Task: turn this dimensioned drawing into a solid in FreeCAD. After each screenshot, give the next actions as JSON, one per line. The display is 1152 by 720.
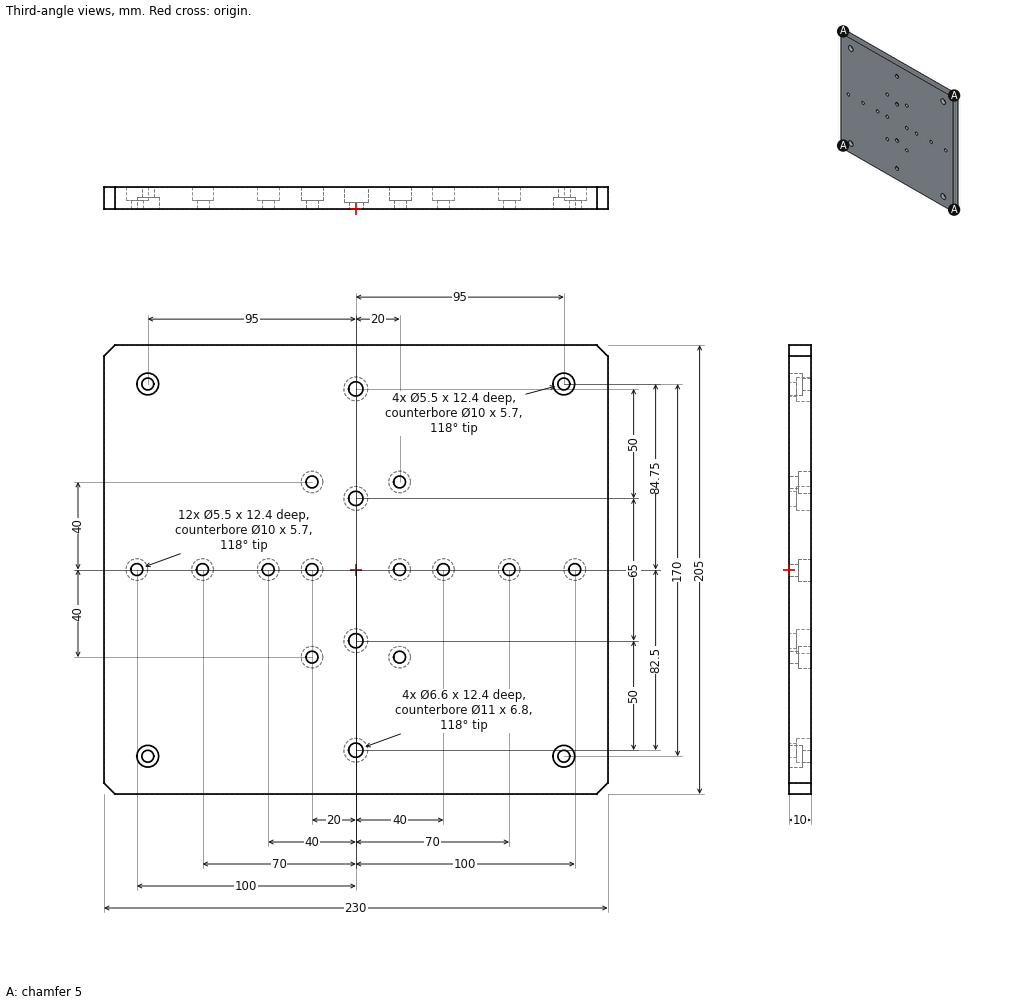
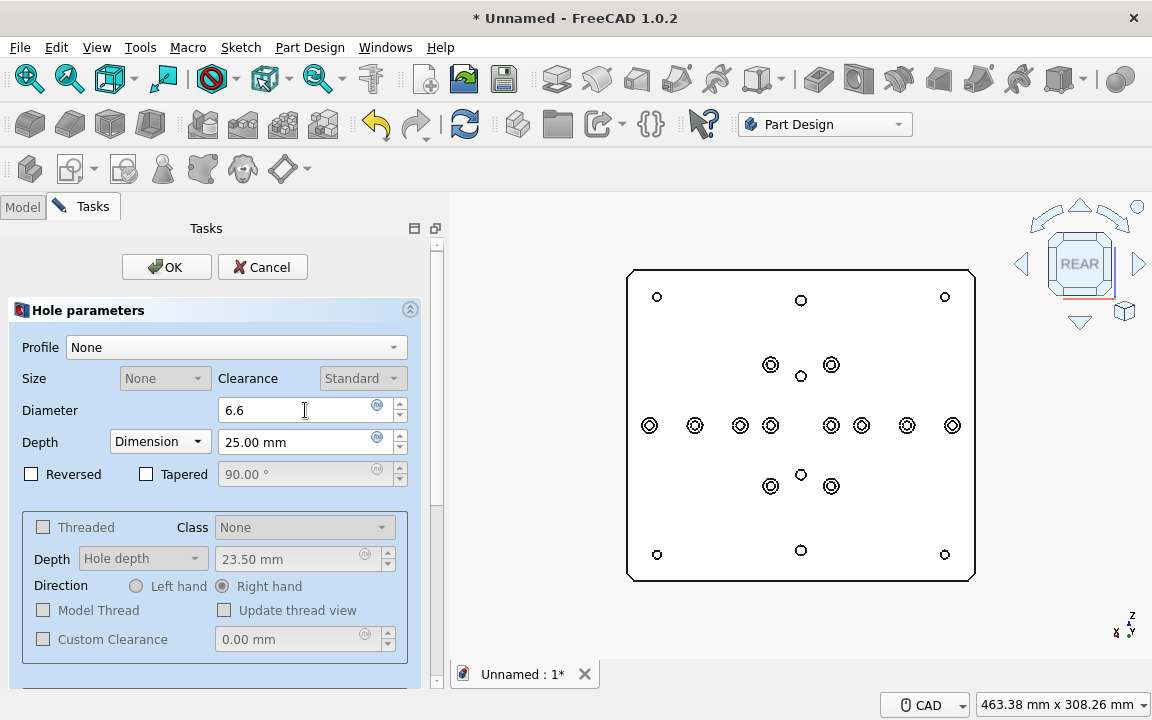
{"action": "triple_click", "coordinate": [305, 442]}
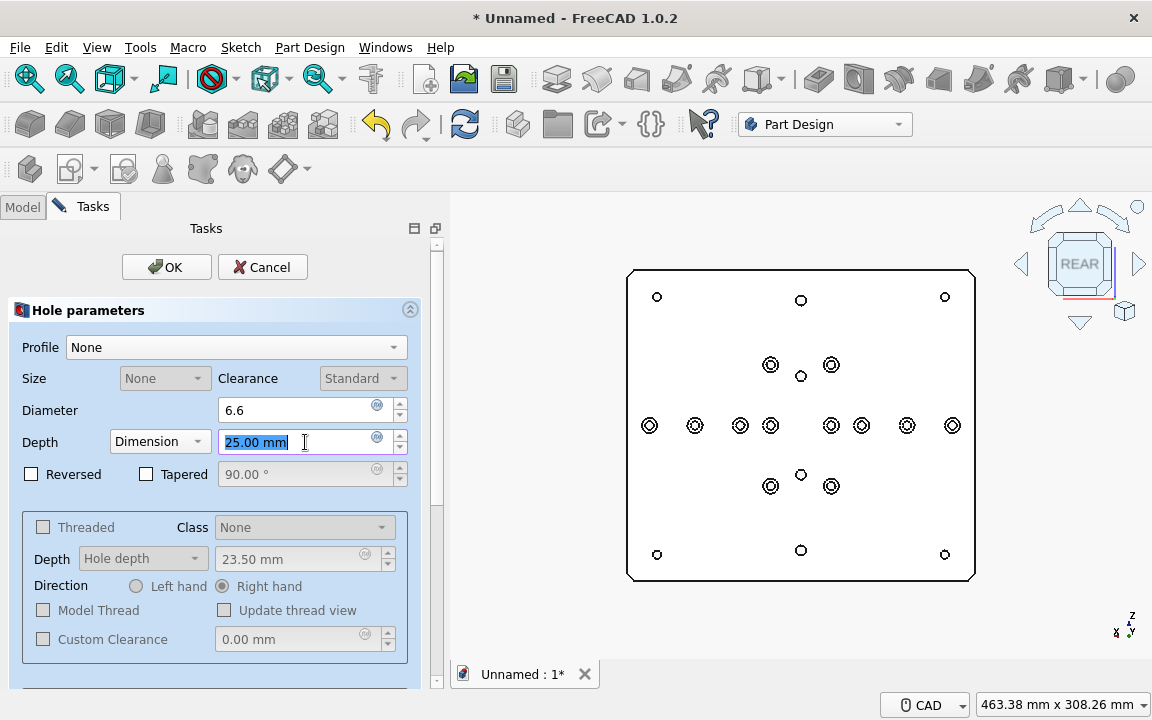
{"action": "type", "text": "12.4"}
{"action": "key", "text": "Tab"}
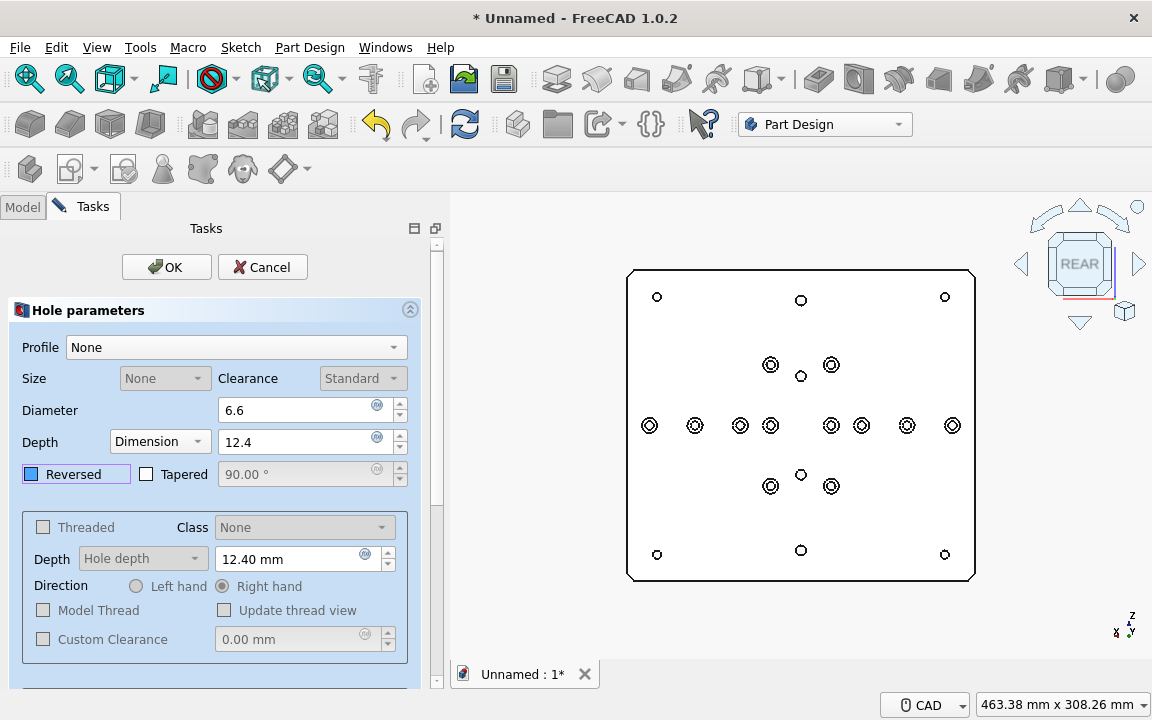
{"action": "scroll", "coordinate": [437, 463], "scroll_direction": "down", "scroll_amount": 2}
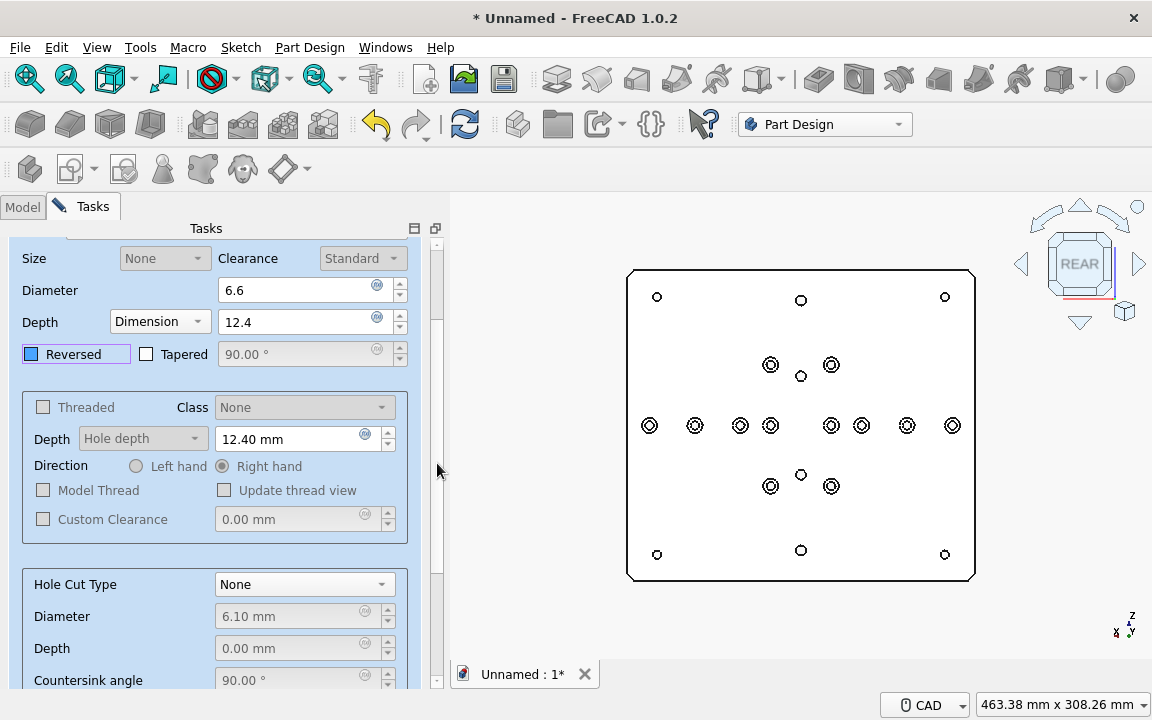
{"action": "left_click", "coordinate": [306, 584]}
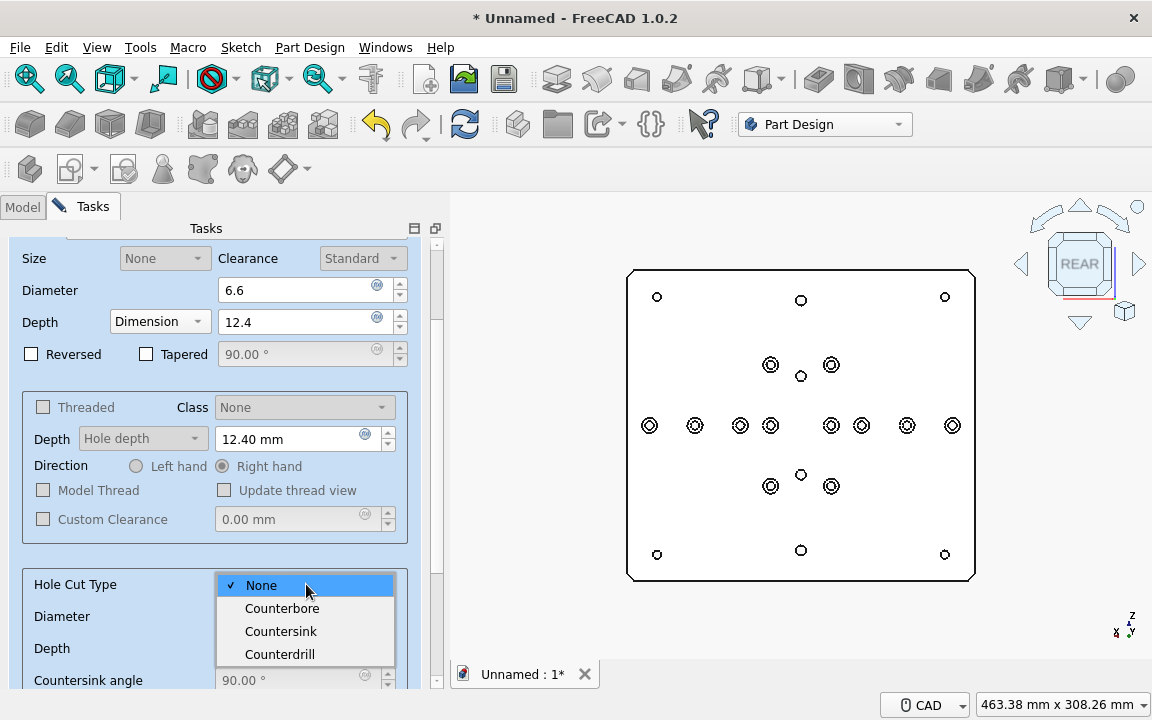
{"action": "left_click", "coordinate": [304, 608]}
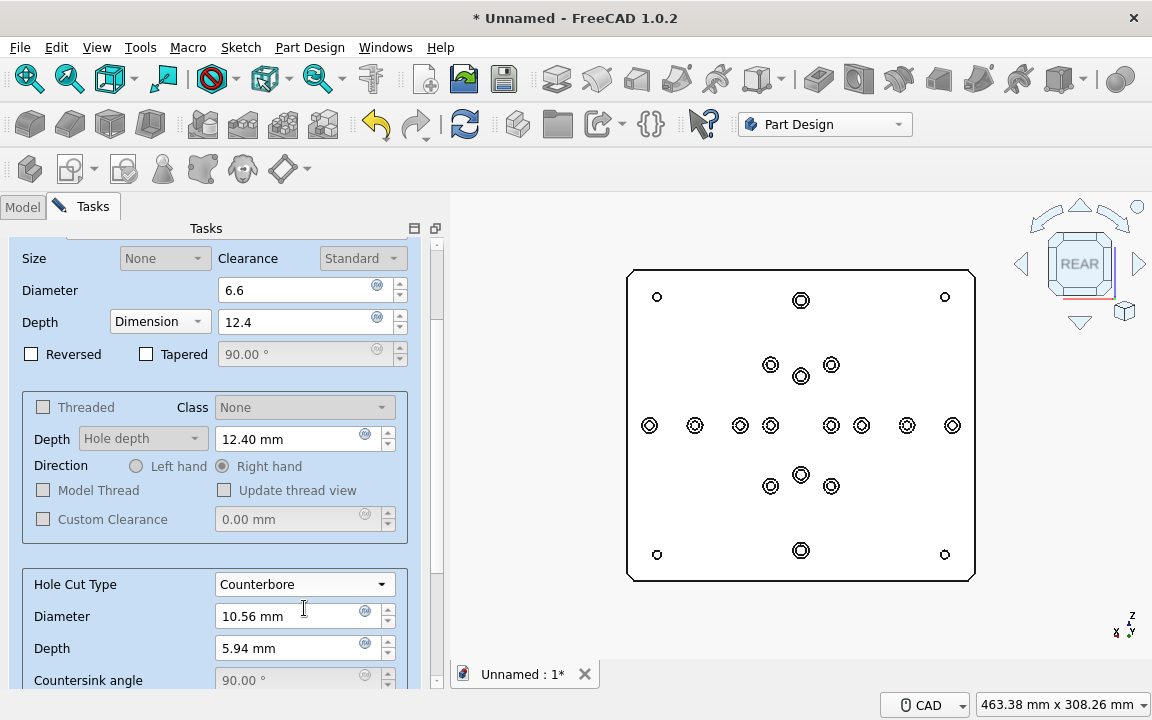
{"action": "triple_click", "coordinate": [298, 616]}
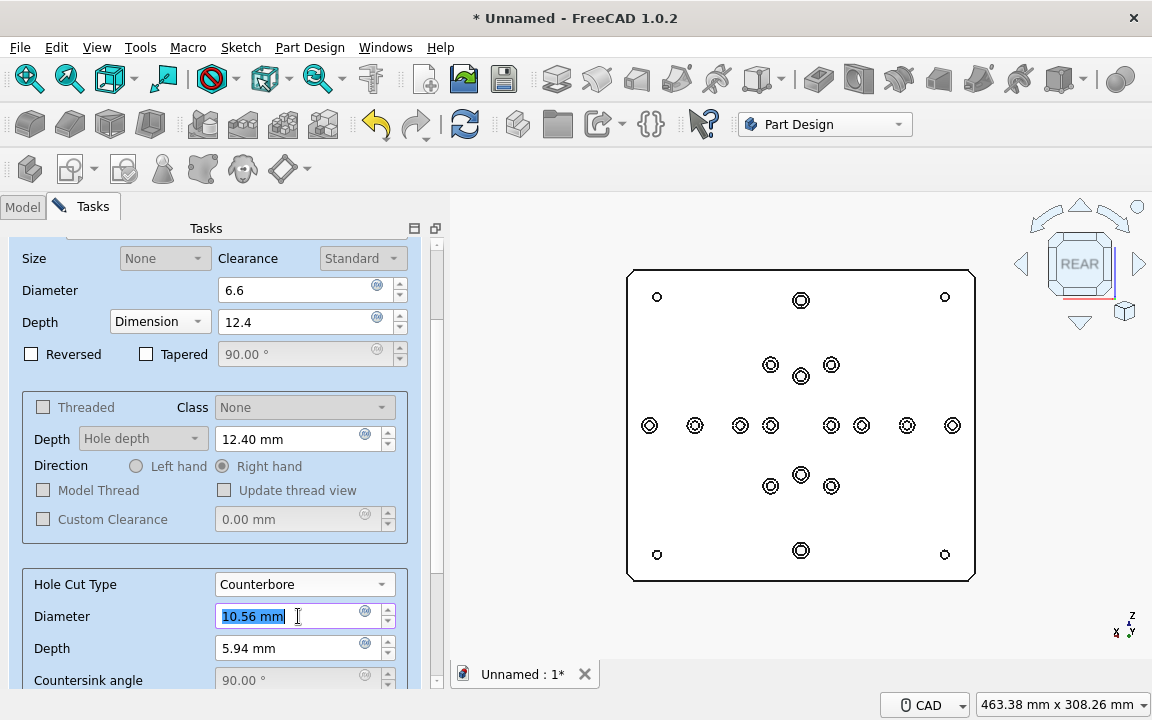
{"action": "type", "text": "11"}
{"action": "key", "text": "Tab"}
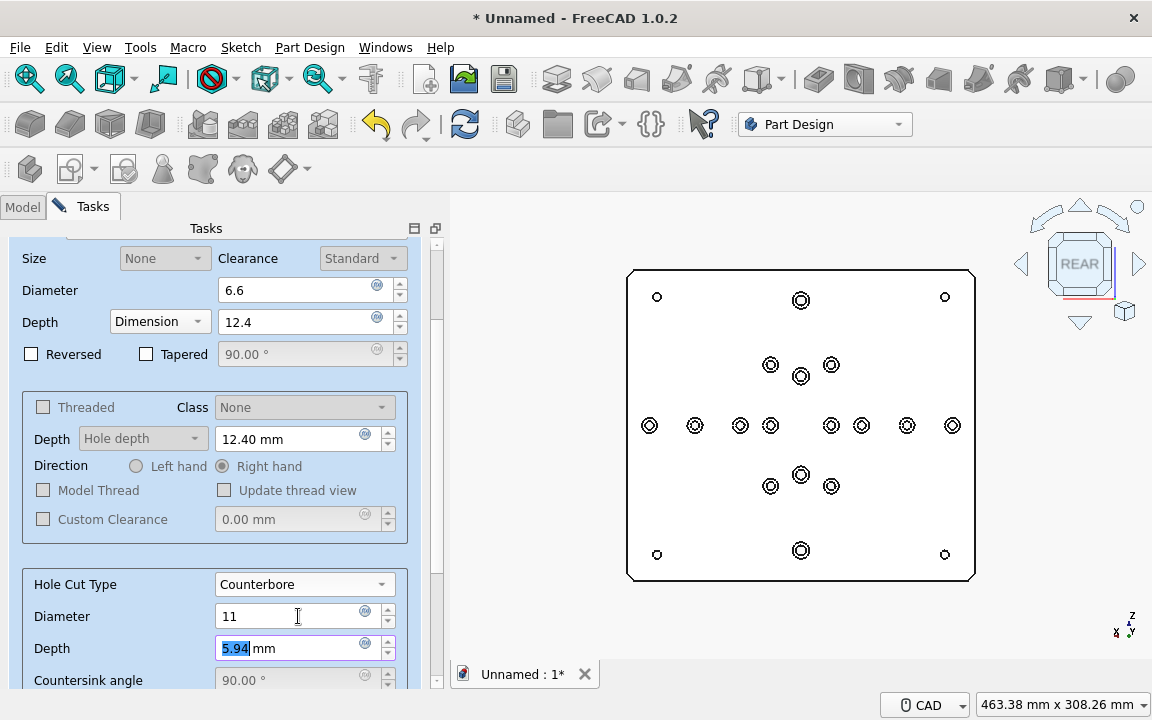
{"action": "type", "text": "6.8"}
{"action": "key", "text": "Tab"}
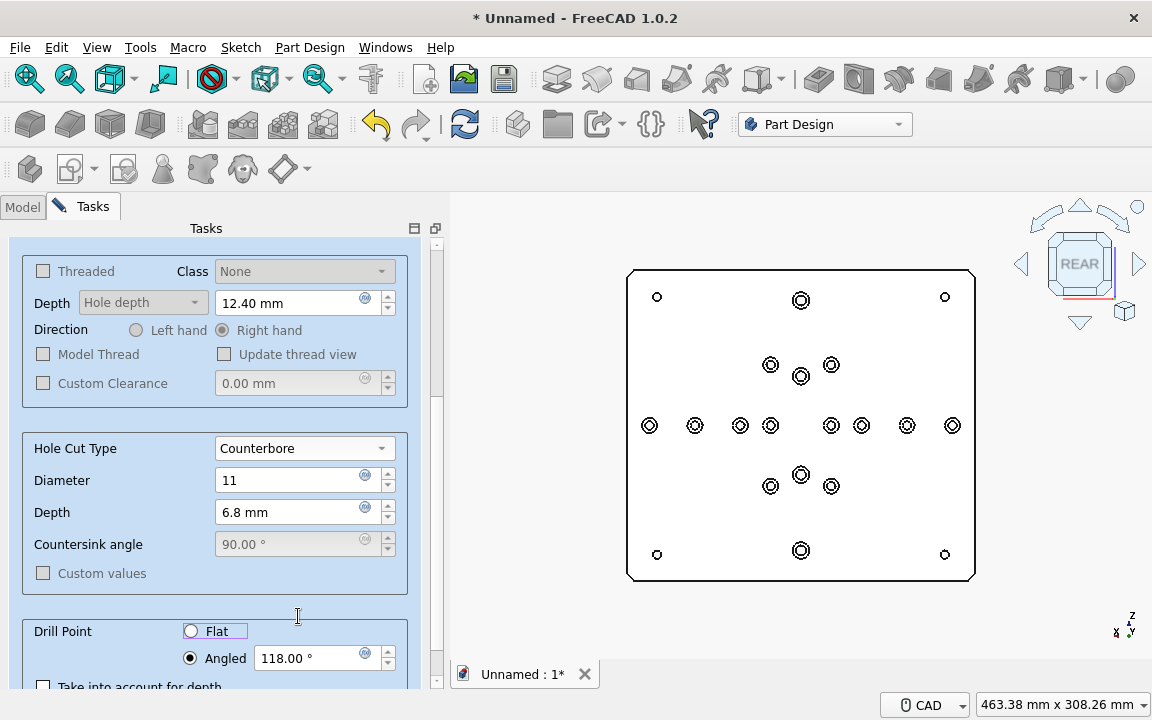
{"action": "scroll", "coordinate": [437, 463], "scroll_direction": "up", "scroll_amount": 6}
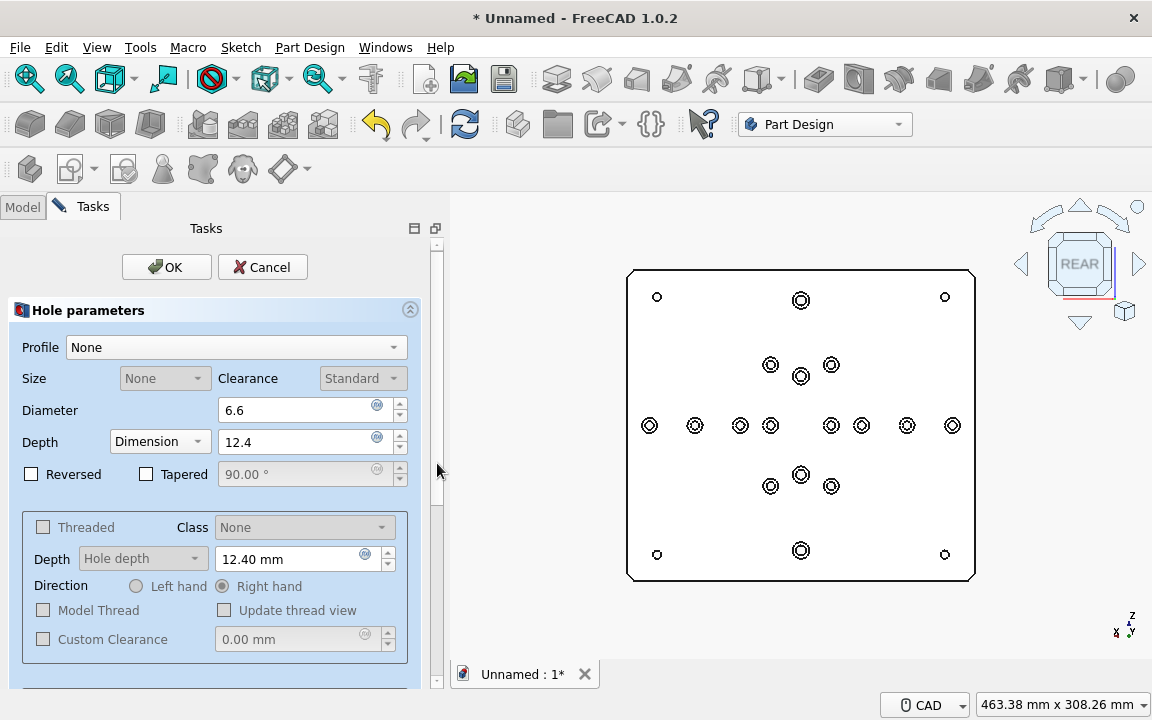
{"action": "left_click", "coordinate": [167, 267]}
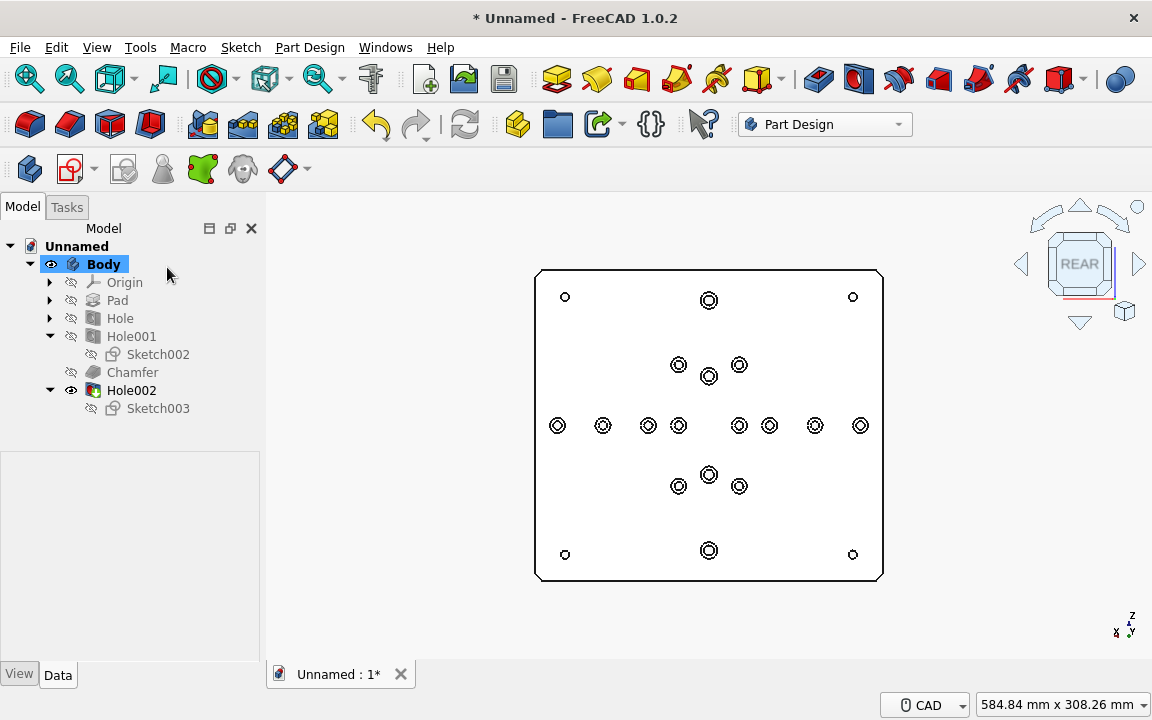
{"action": "key", "text": "0"}